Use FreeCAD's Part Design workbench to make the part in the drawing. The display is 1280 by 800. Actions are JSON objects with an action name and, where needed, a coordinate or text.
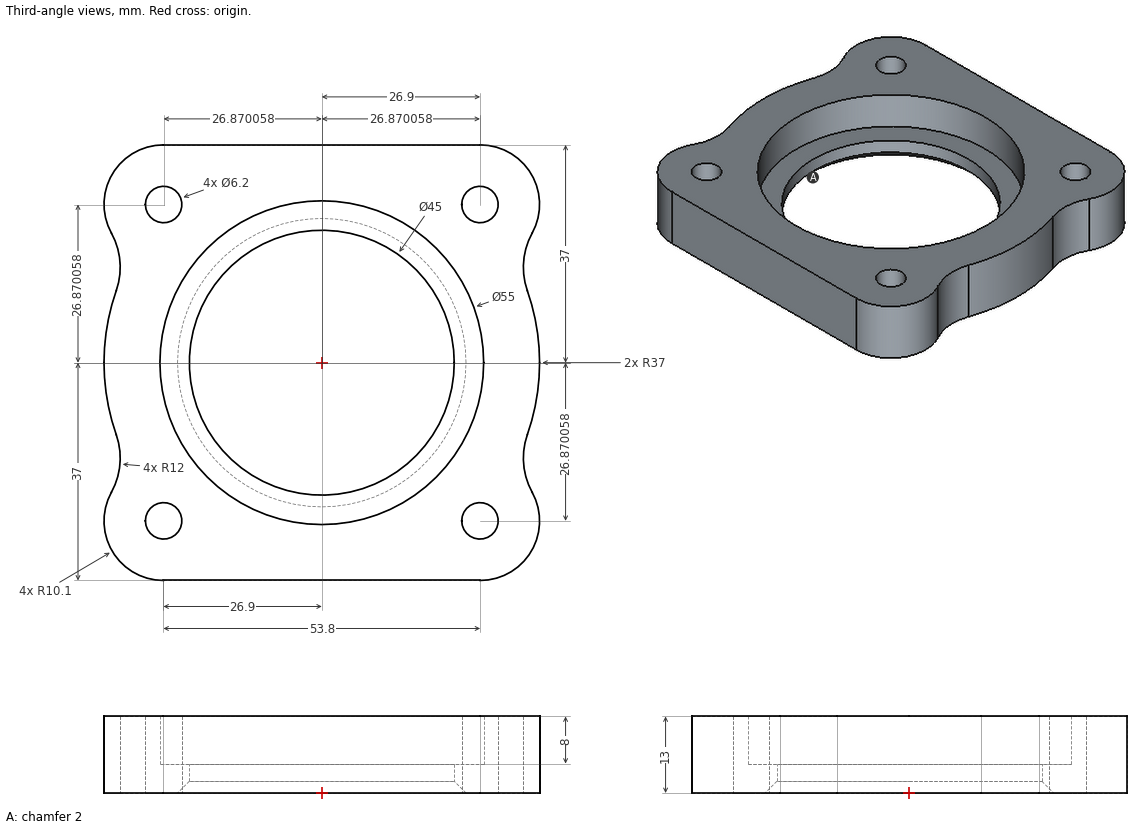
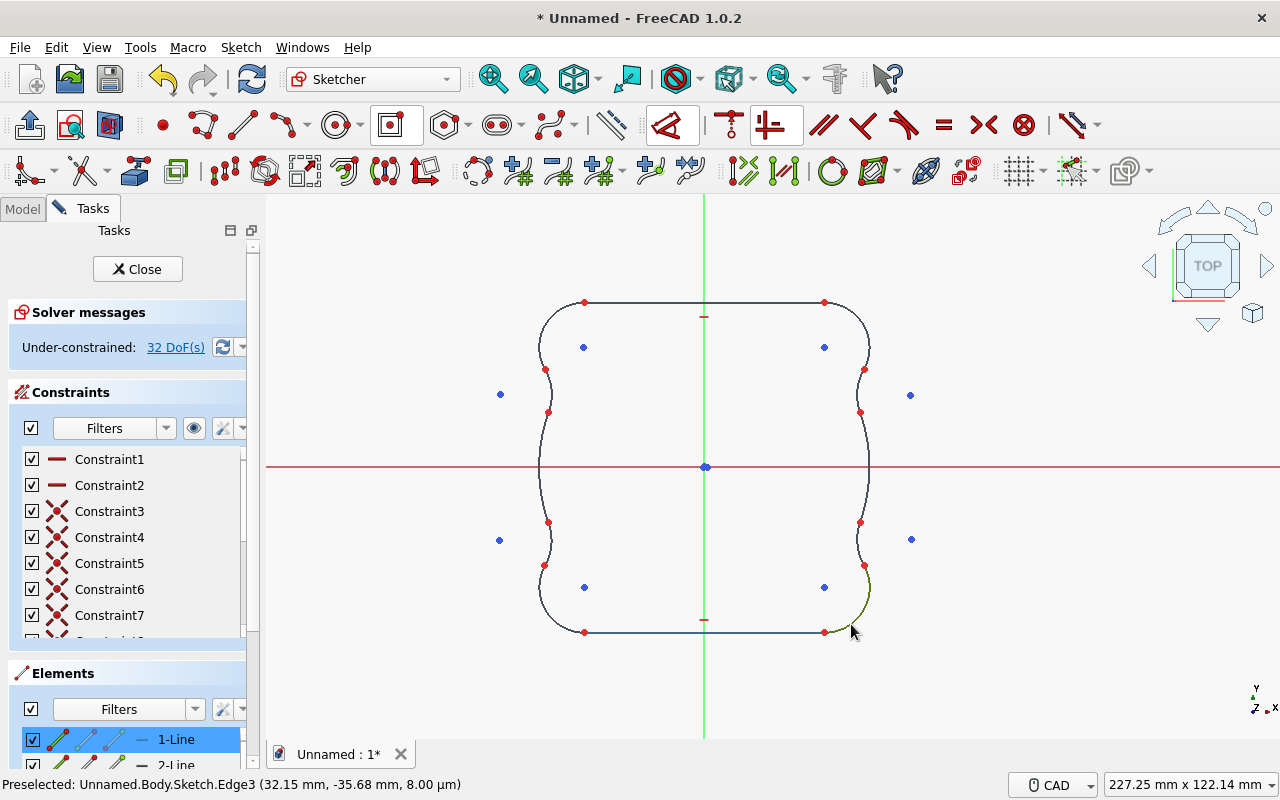
{"action": "key", "text": "t"}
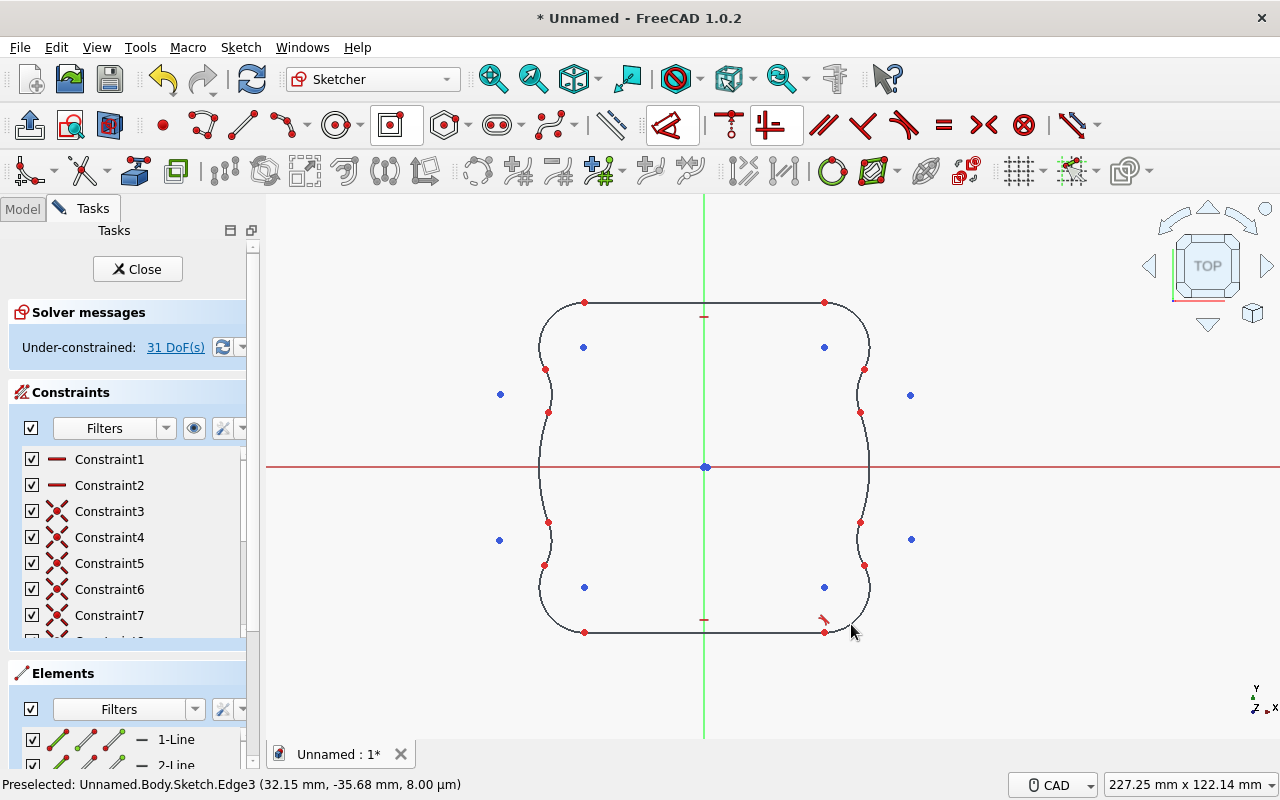
{"action": "left_click", "coordinate": [656, 633]}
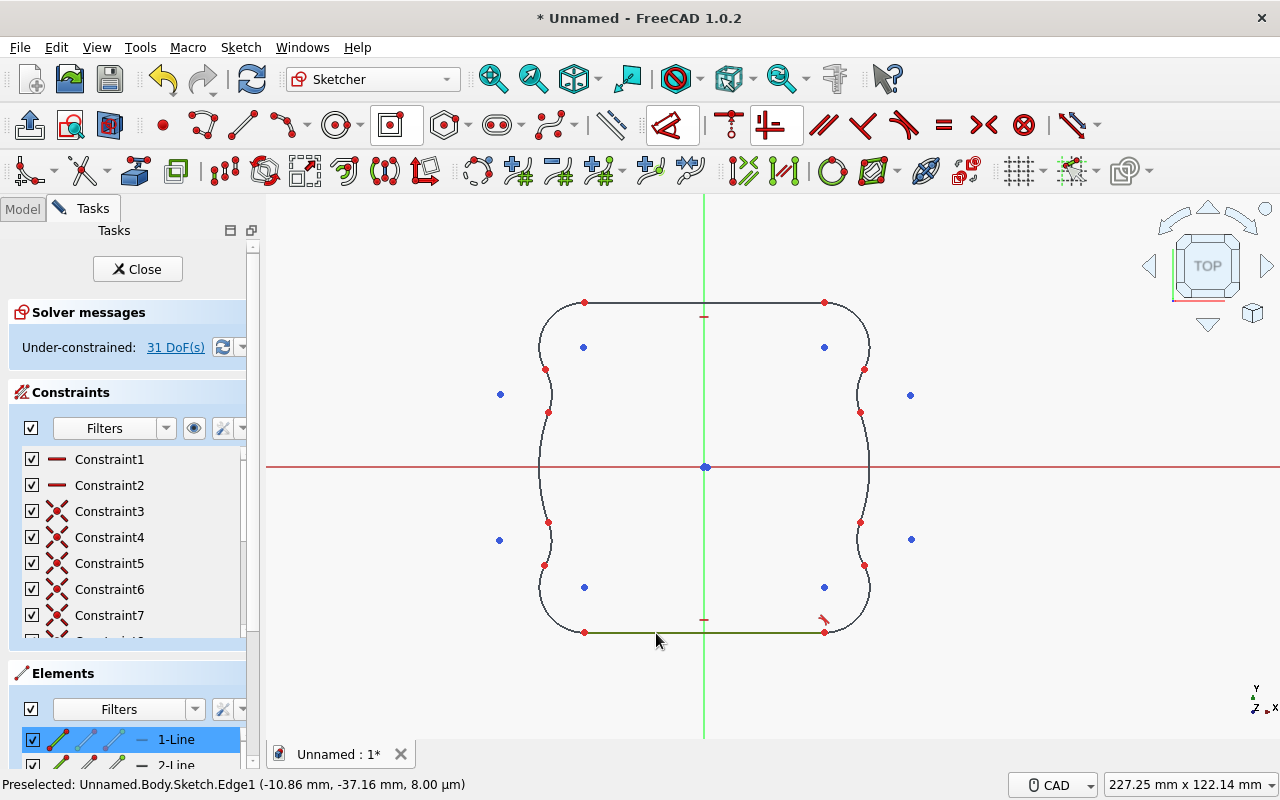
{"action": "left_click", "coordinate": [540, 593]}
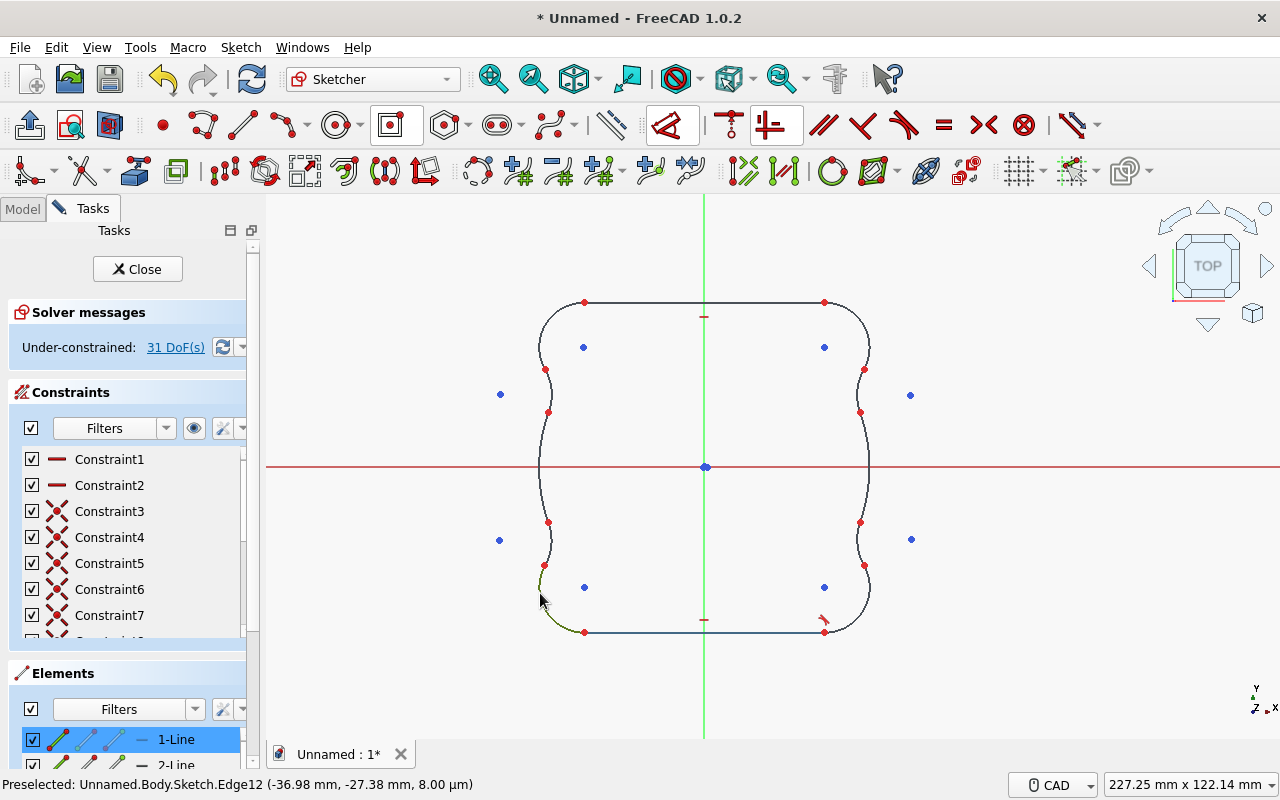
{"action": "key", "text": "t"}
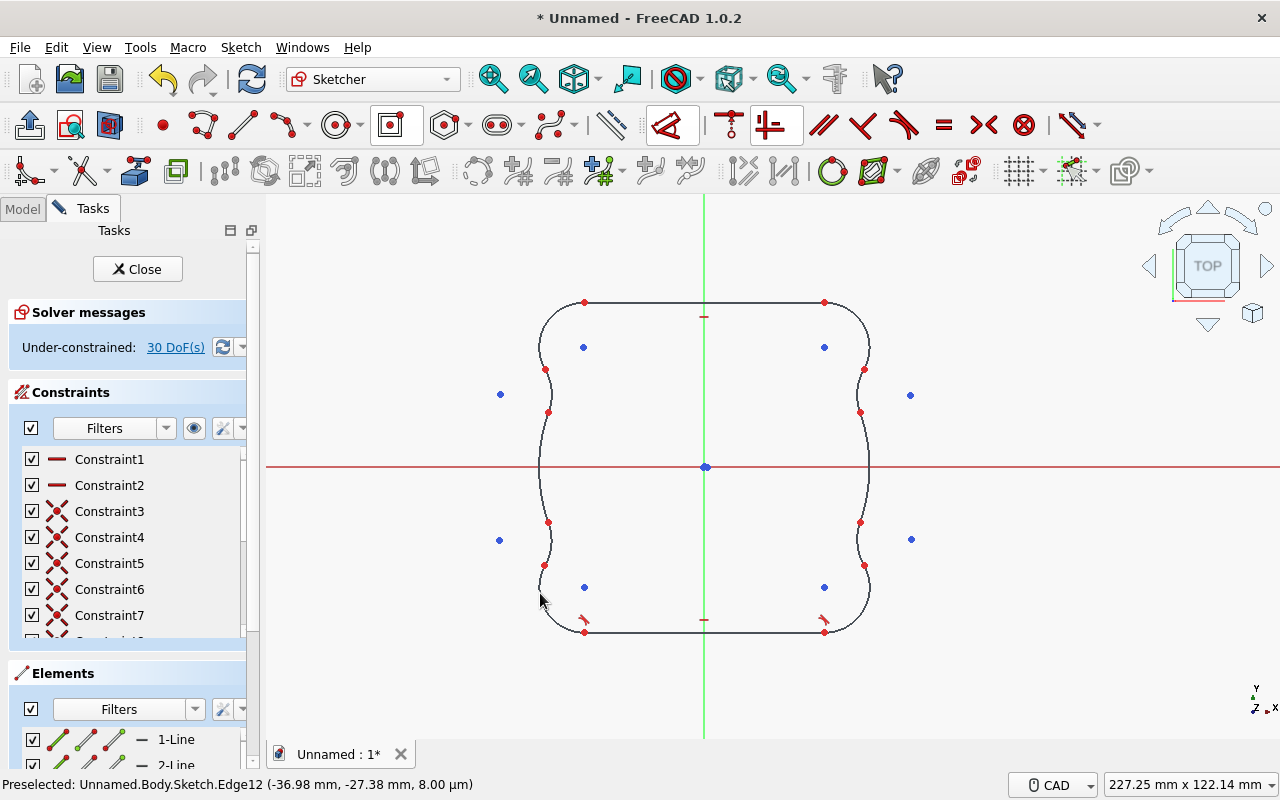
{"action": "left_click", "coordinate": [753, 303]}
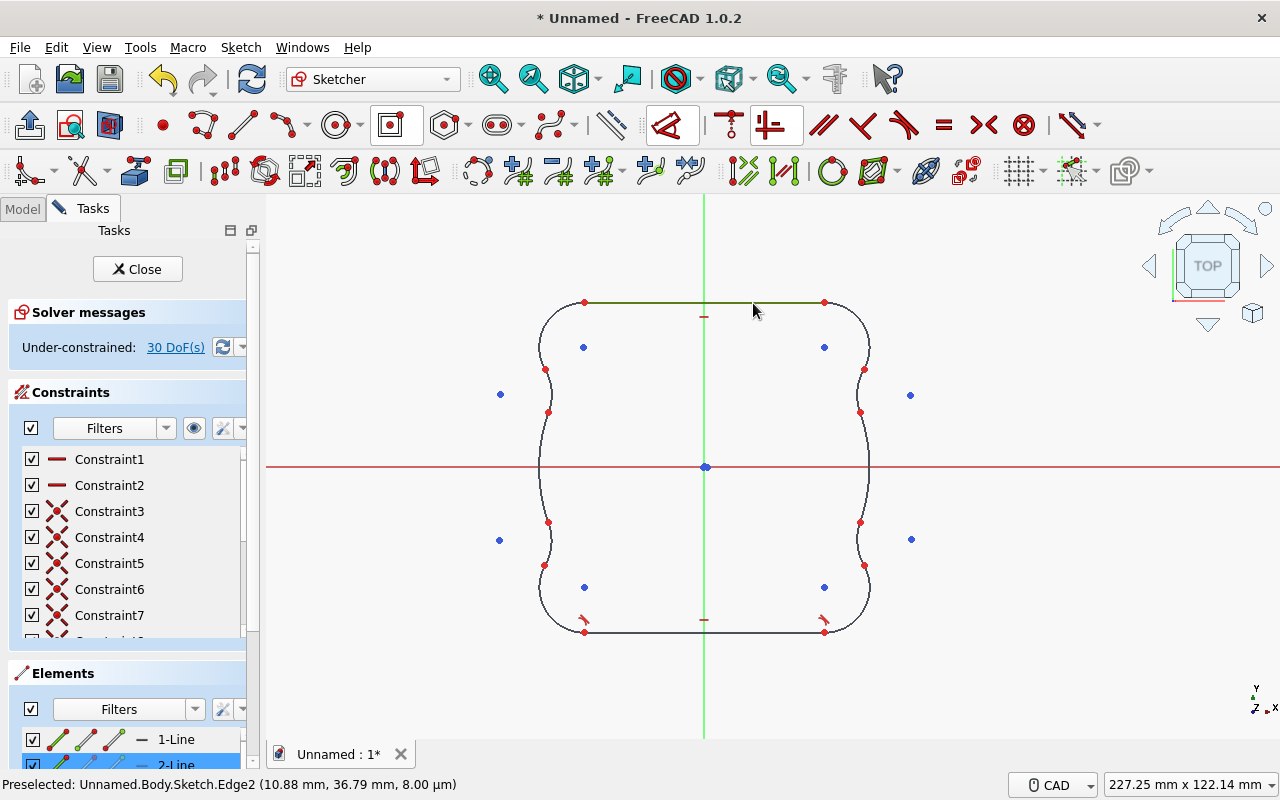
{"action": "left_click", "coordinate": [869, 342]}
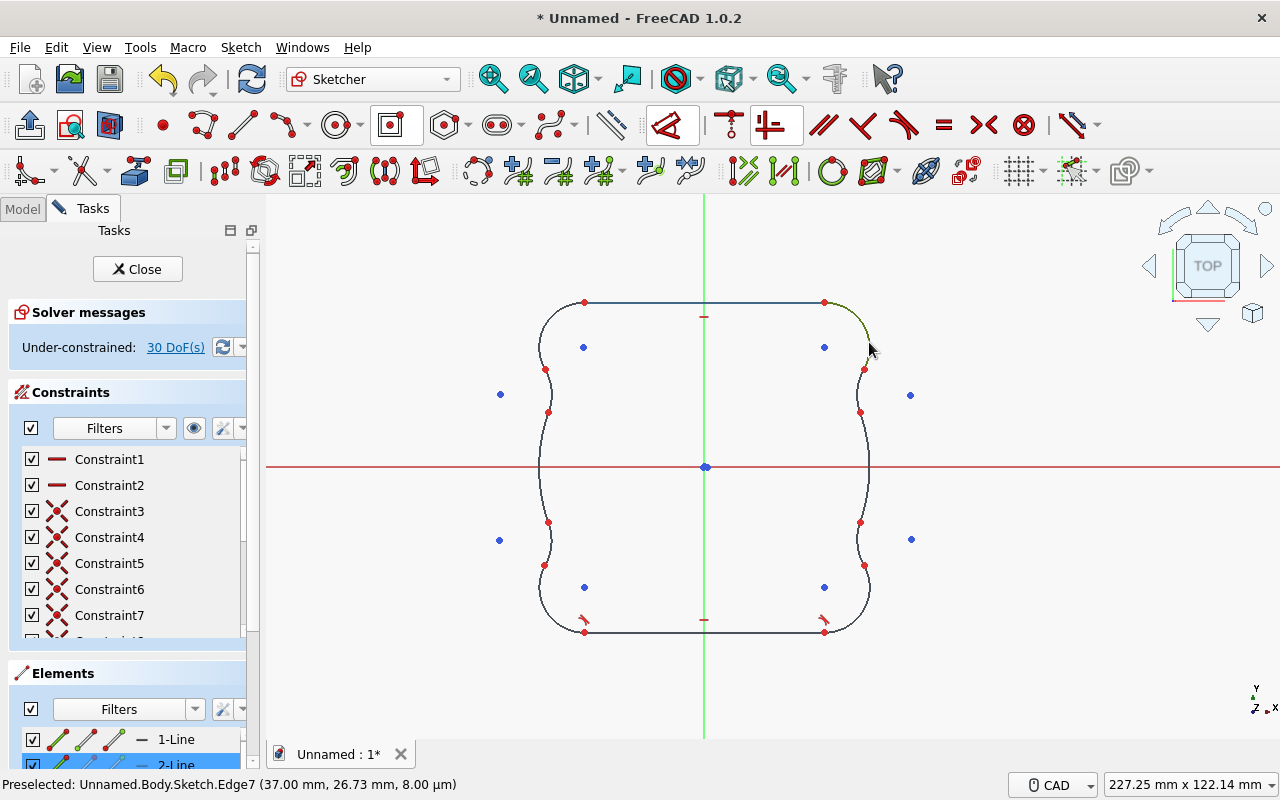
{"action": "left_click", "coordinate": [904, 126]}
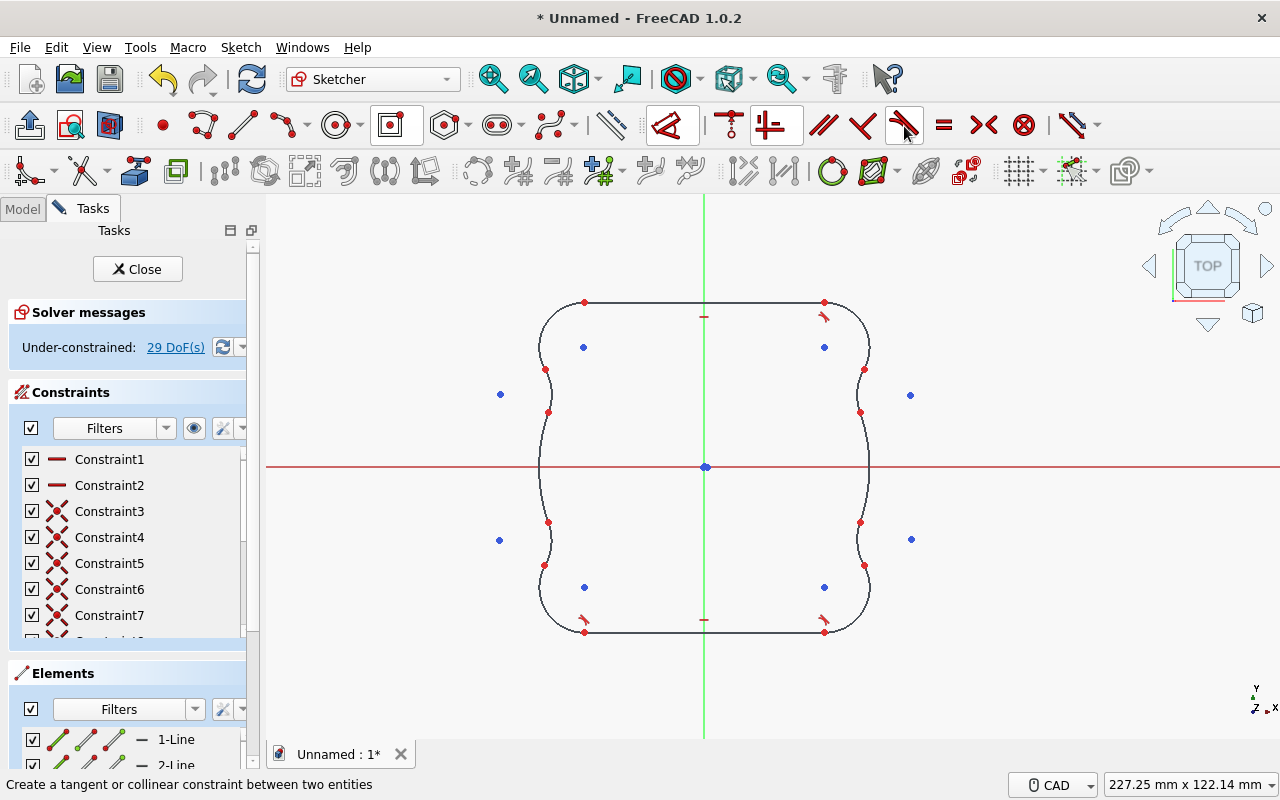
{"action": "left_click", "coordinate": [753, 303]}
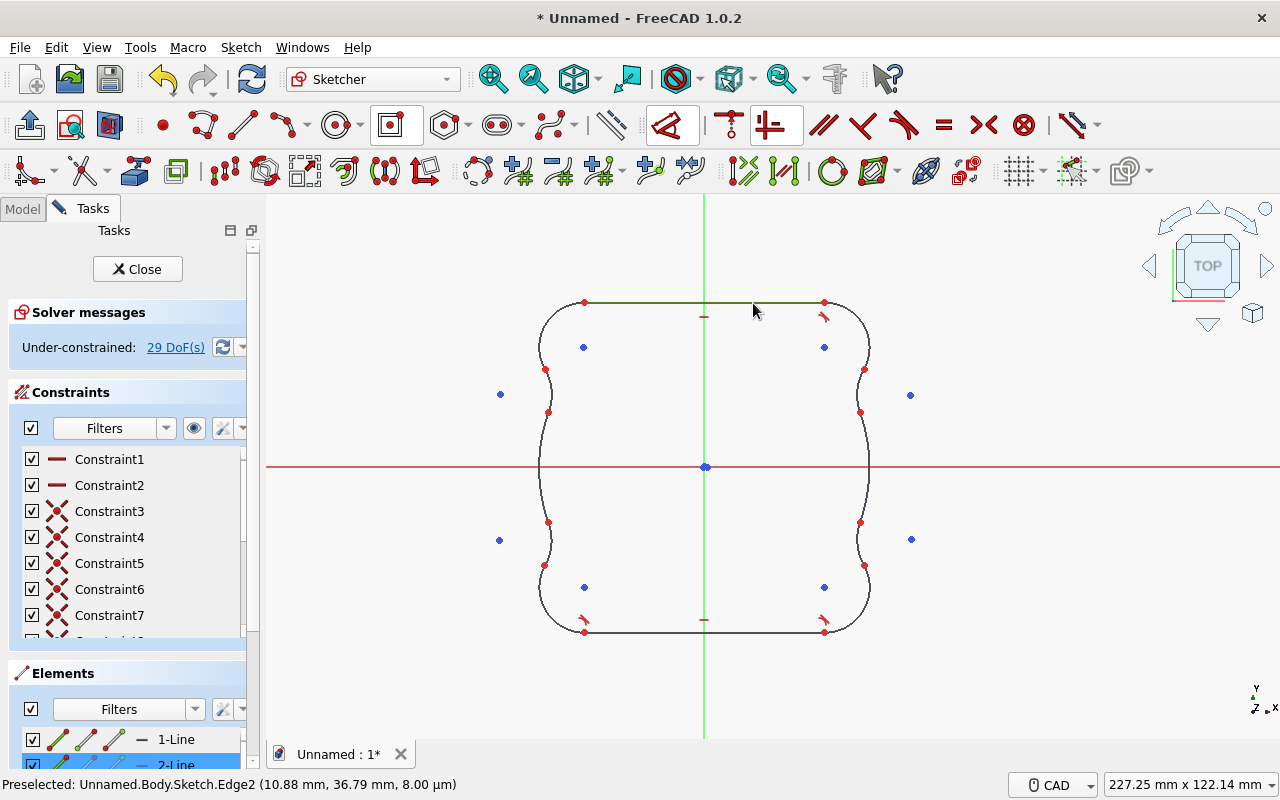
{"action": "left_click", "coordinate": [558, 311]}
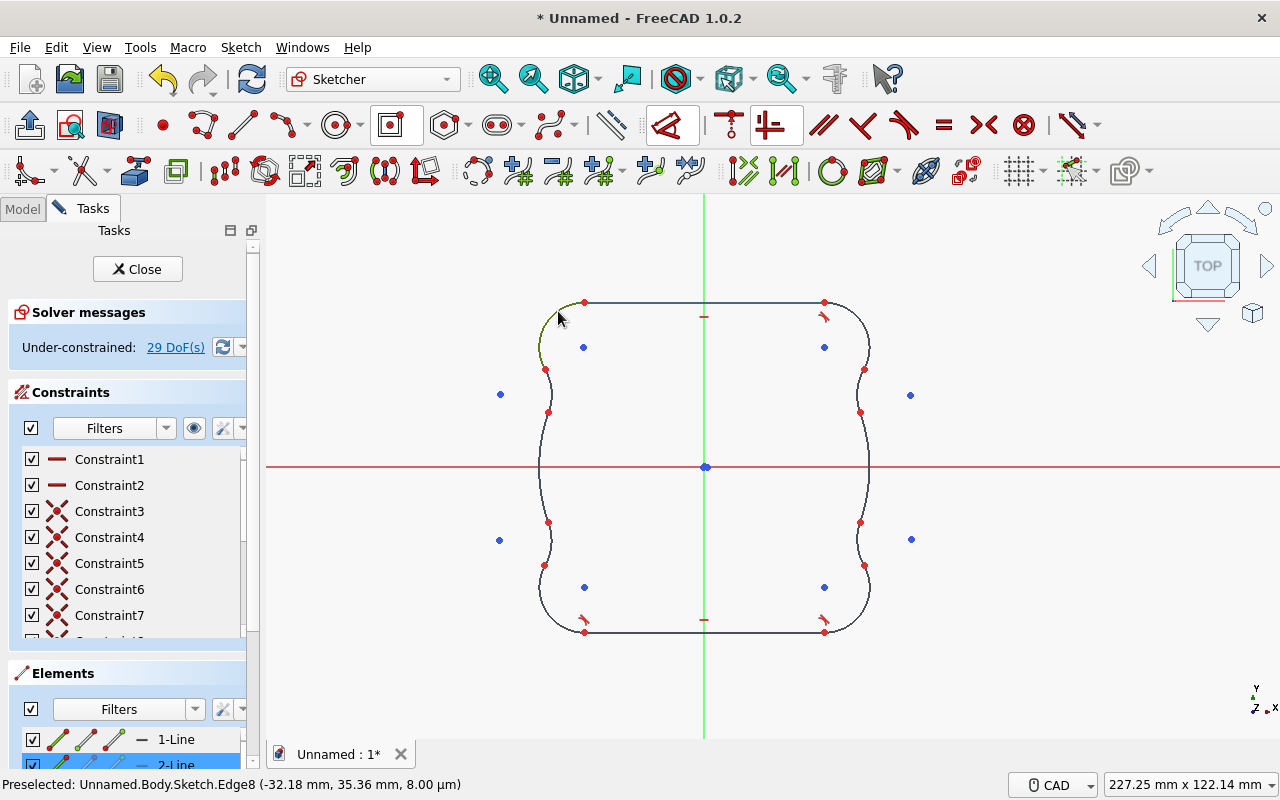
{"action": "key", "text": "t"}